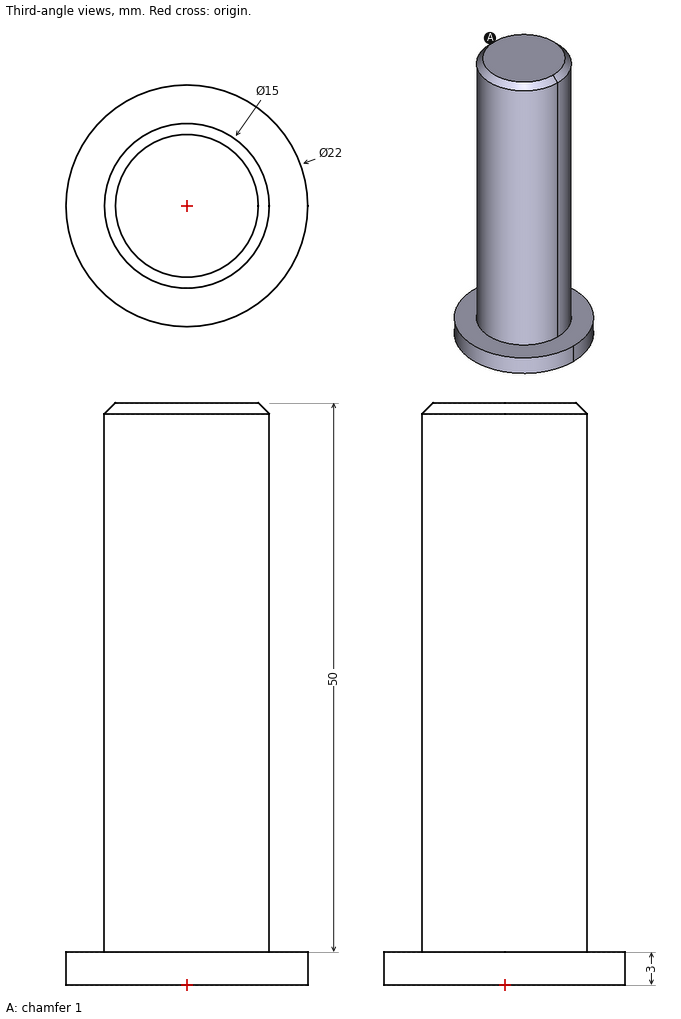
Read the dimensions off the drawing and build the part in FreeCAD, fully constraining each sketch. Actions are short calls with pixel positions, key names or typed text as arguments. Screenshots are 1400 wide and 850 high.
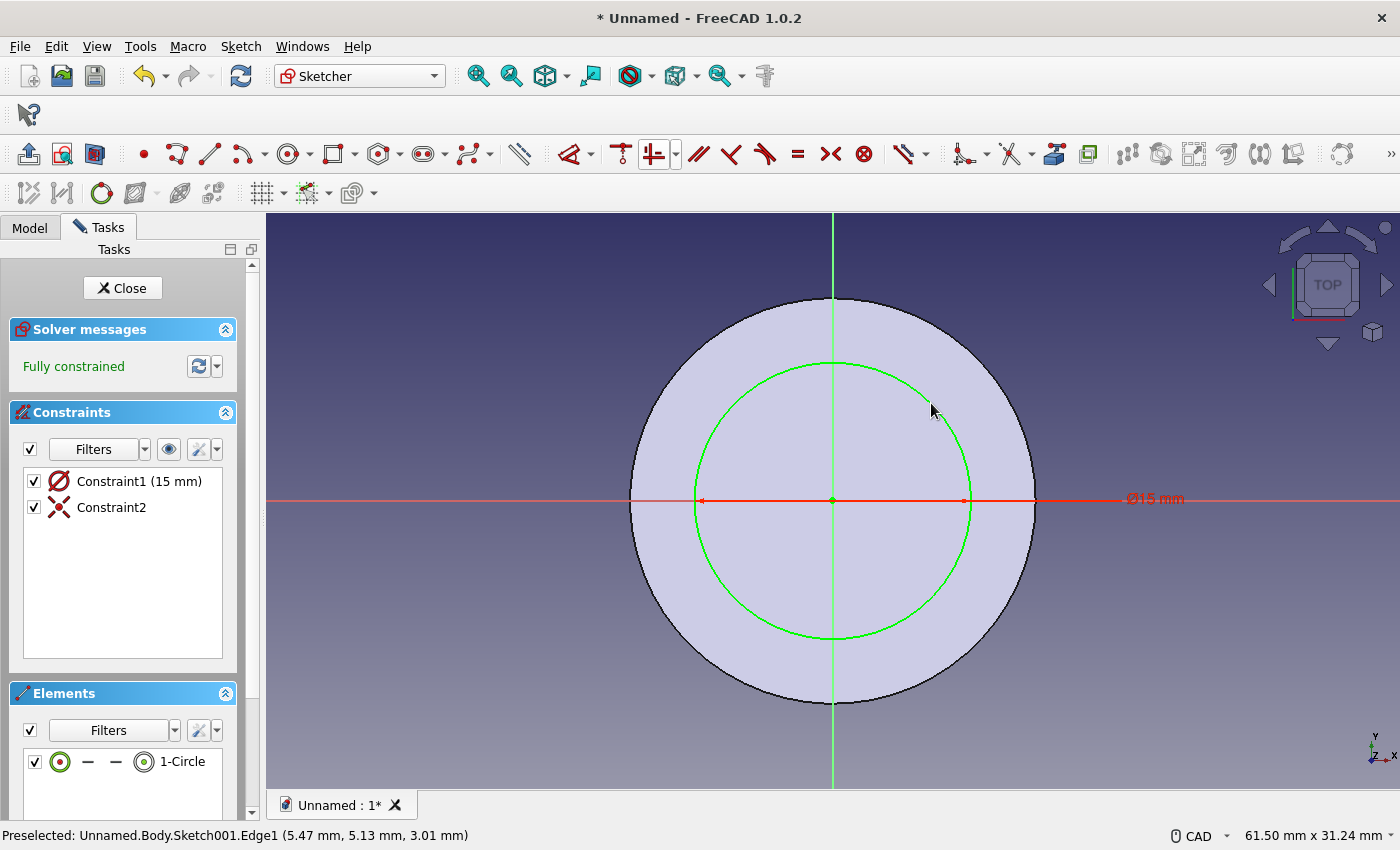
click(123, 288)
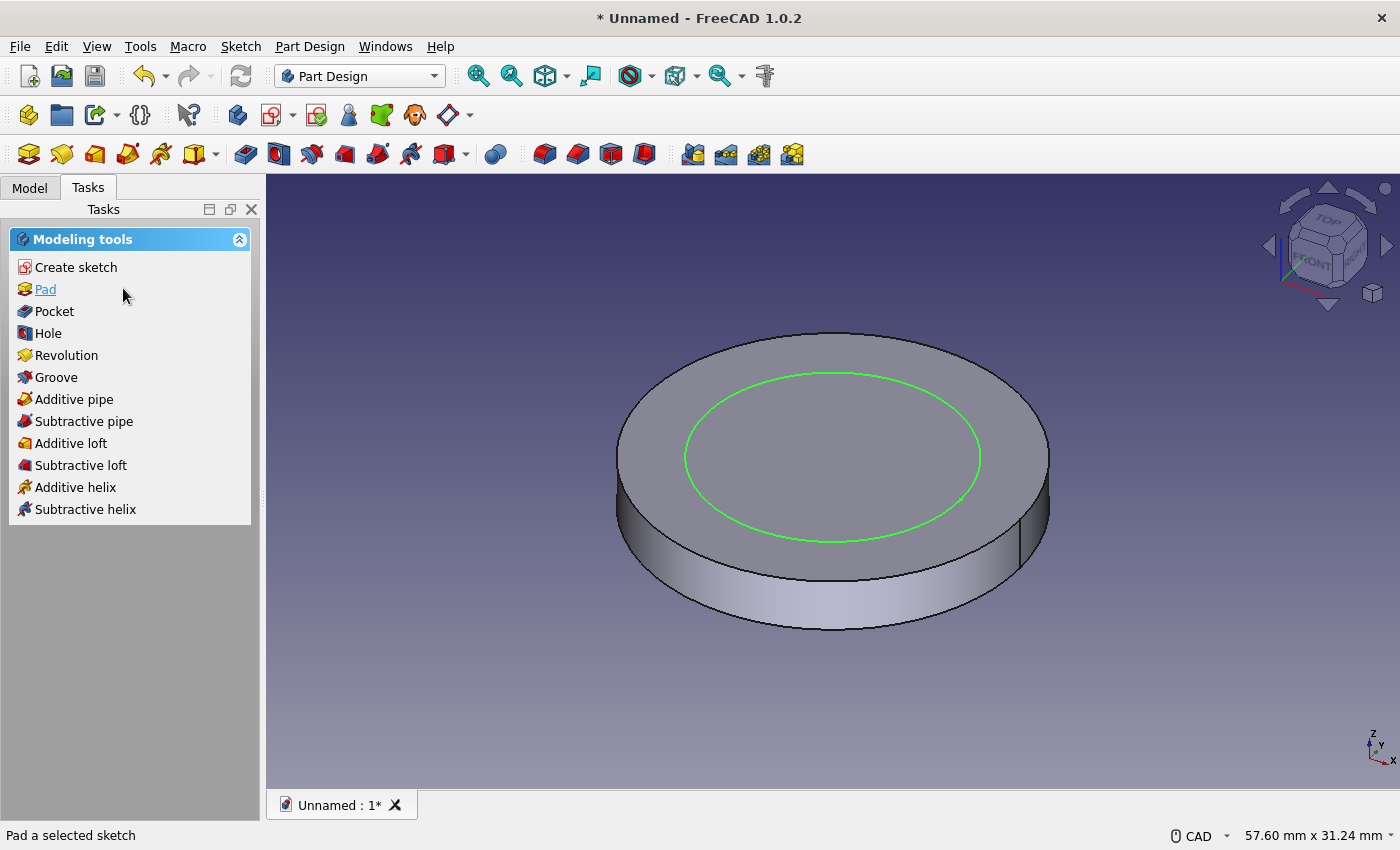
click(29, 154)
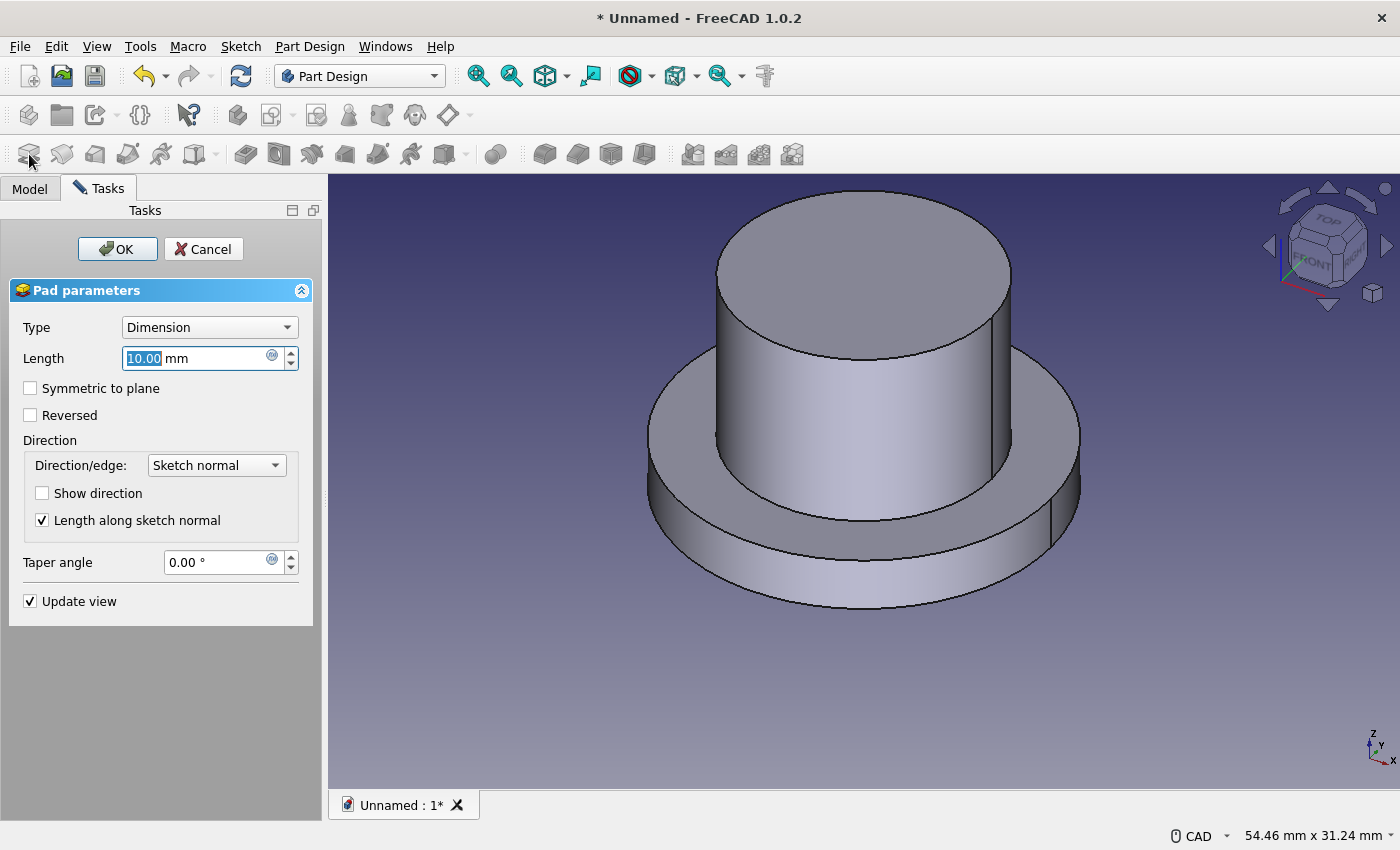
text(50)
key(Tab)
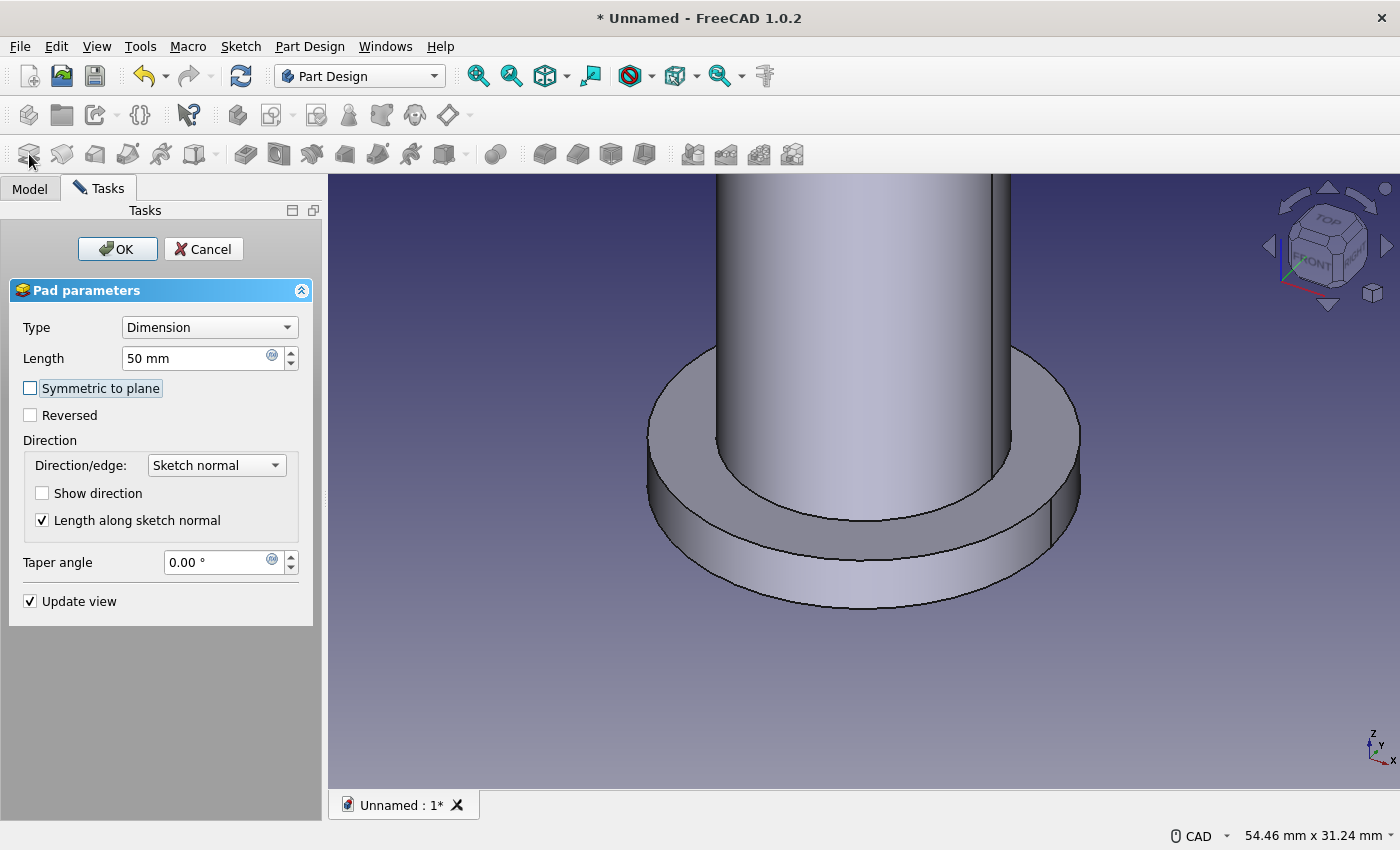
click(118, 249)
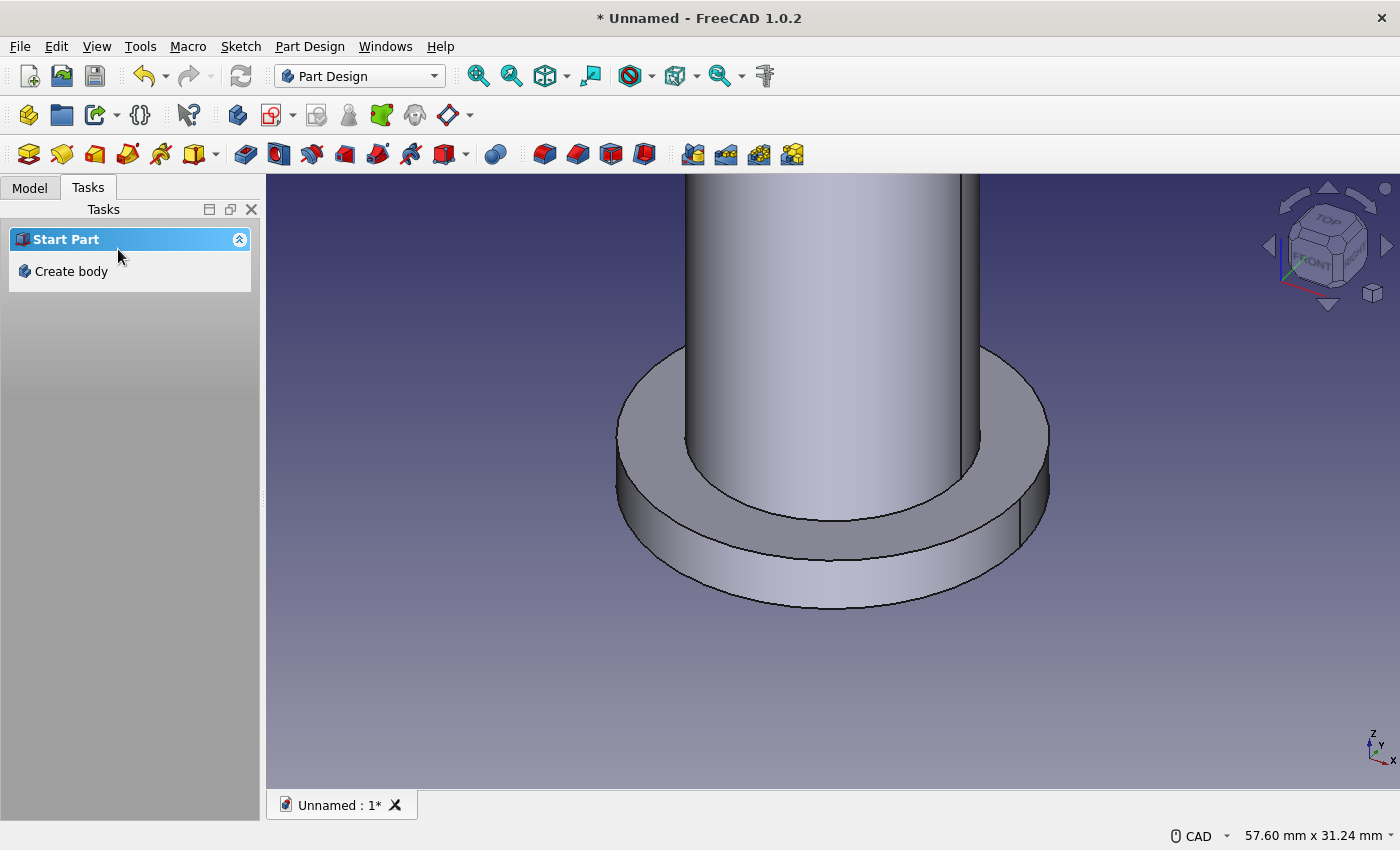
click(479, 76)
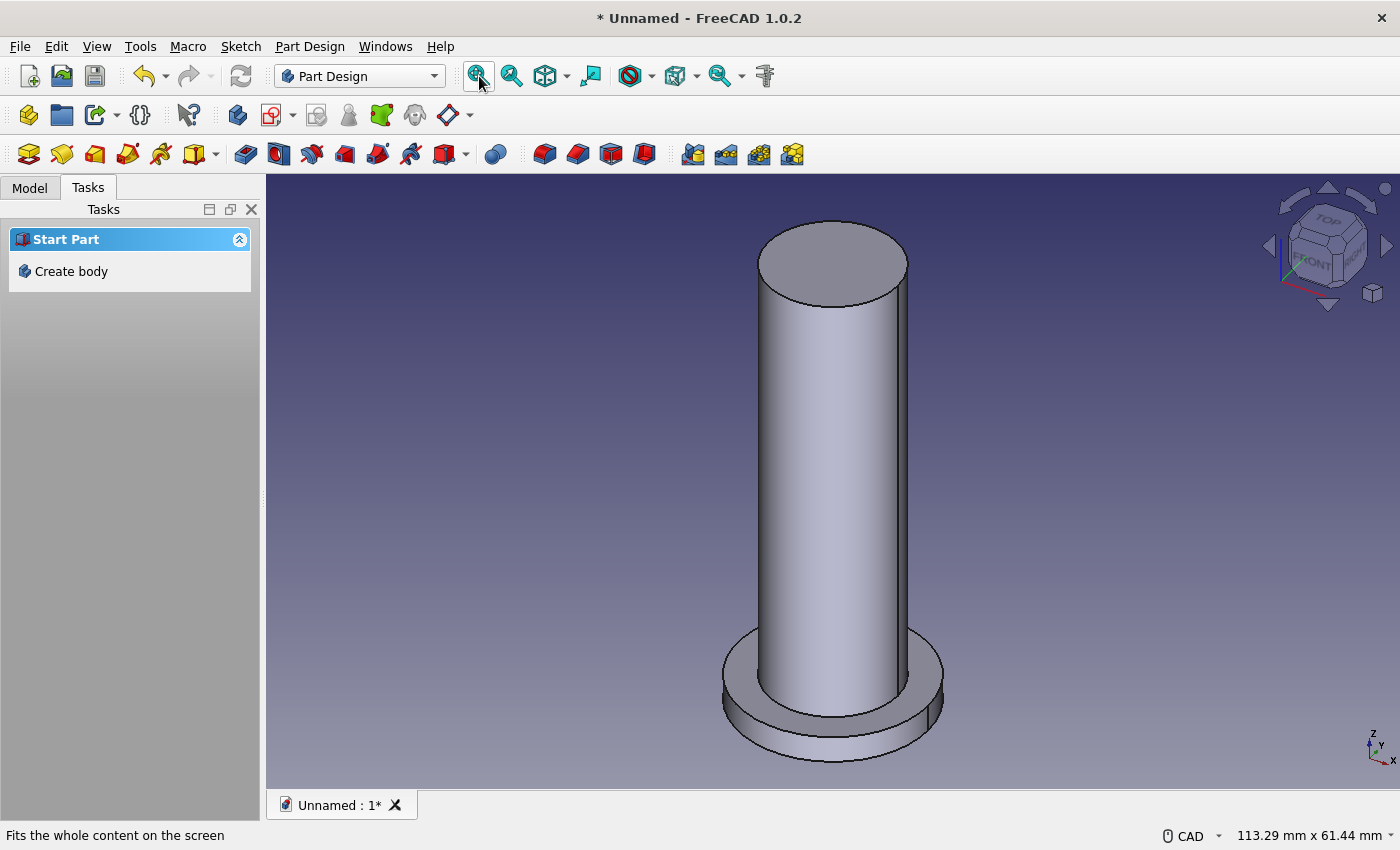
click(758, 268)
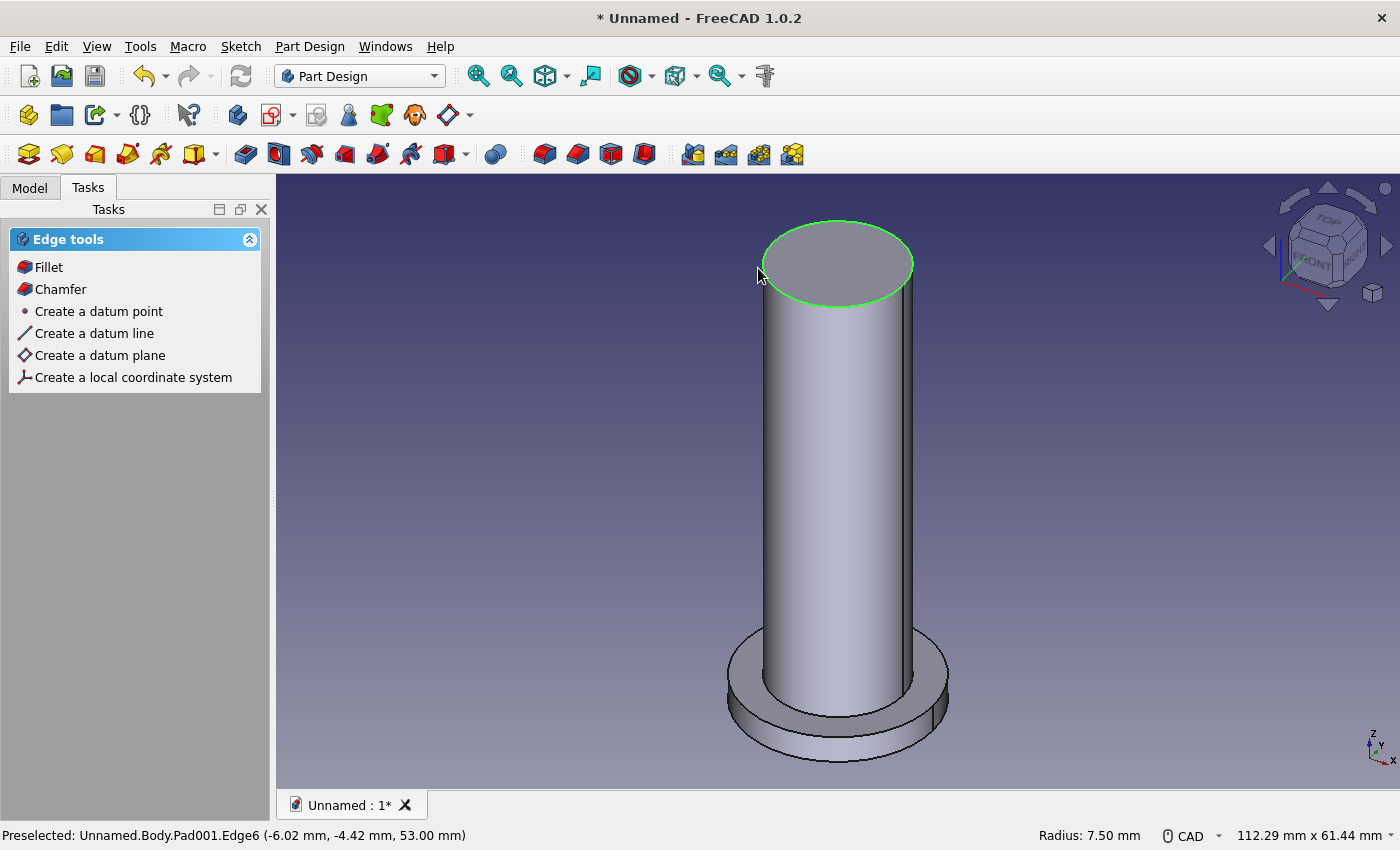
click(578, 154)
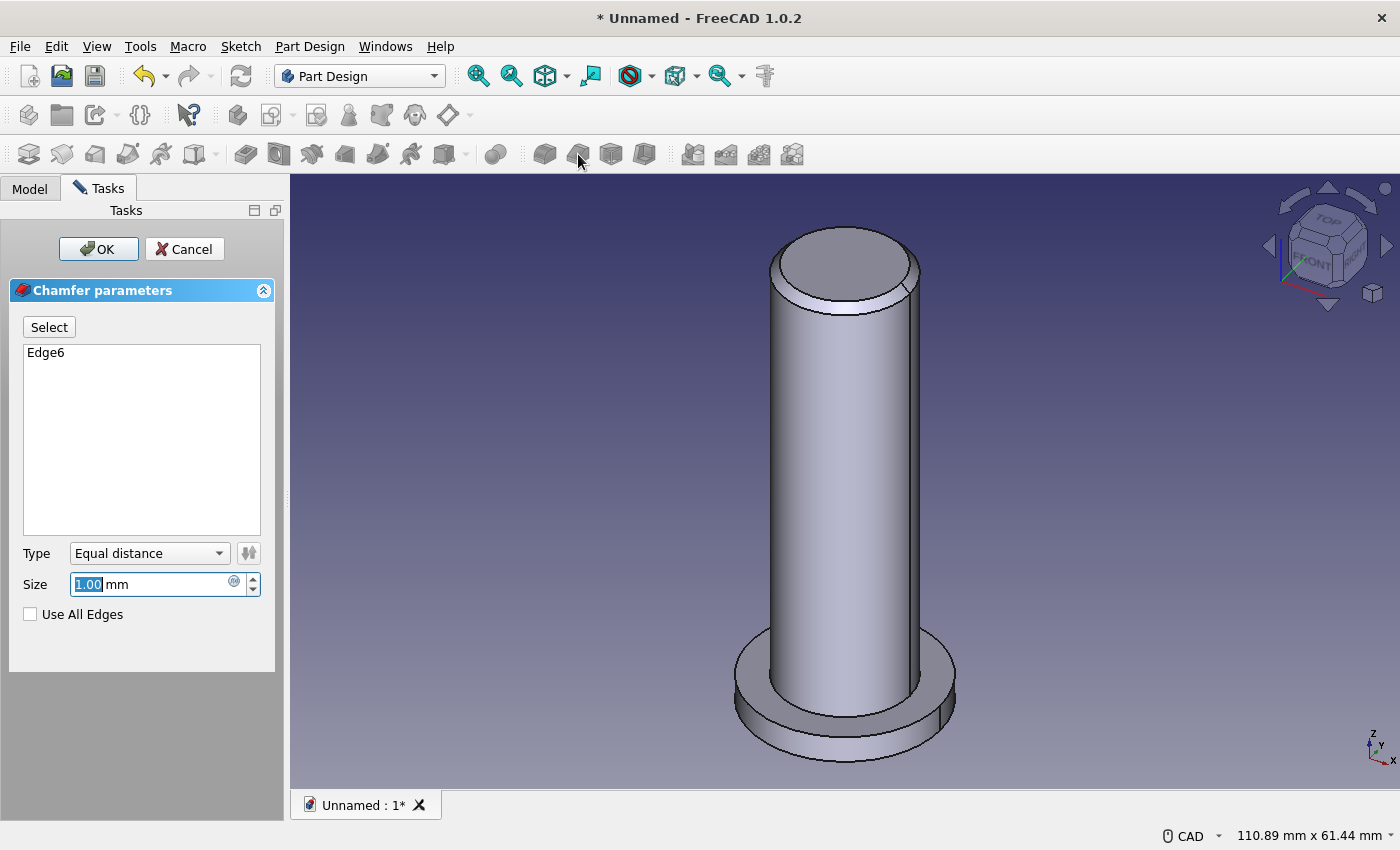
text(1)
key(Tab)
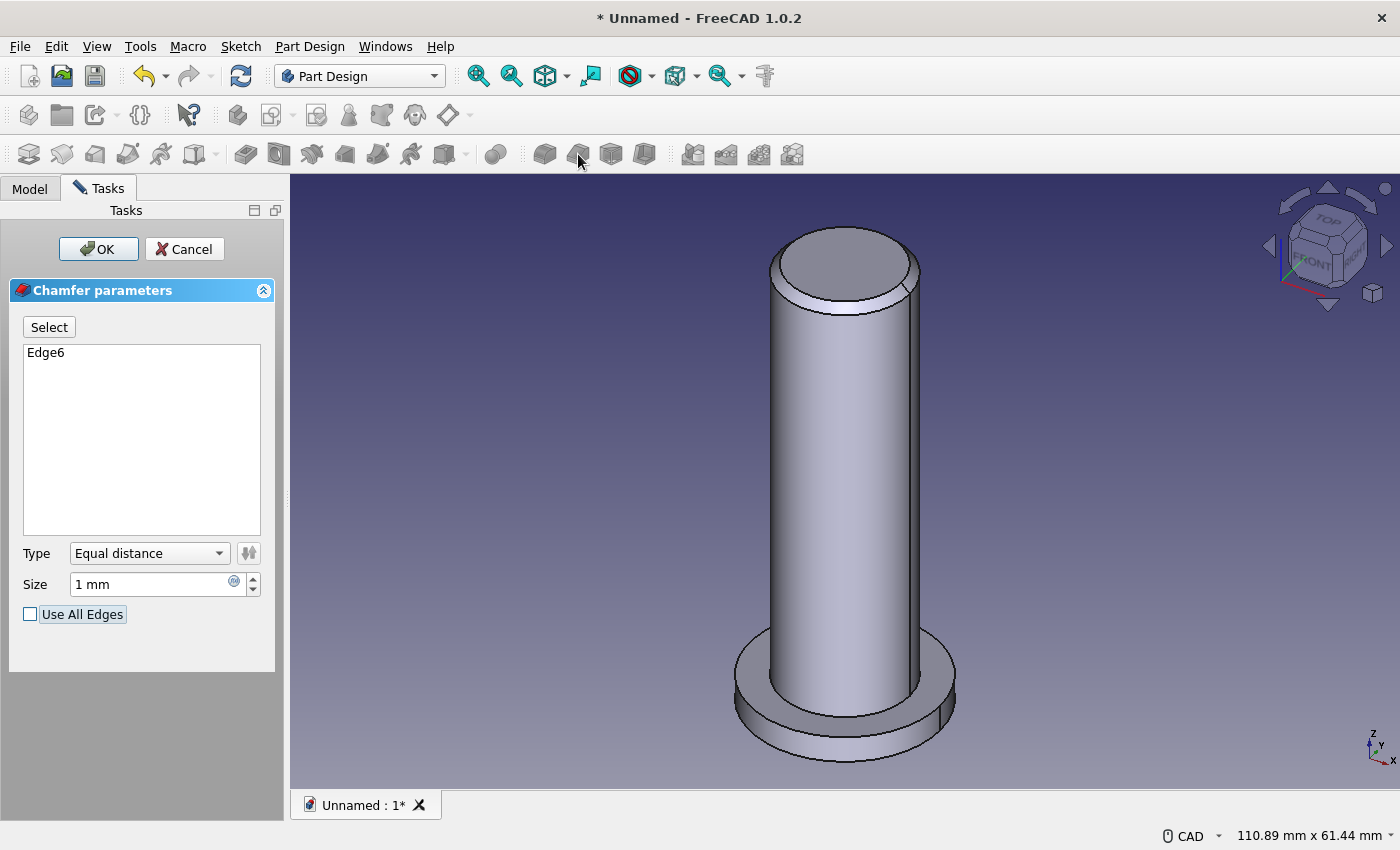
click(99, 249)